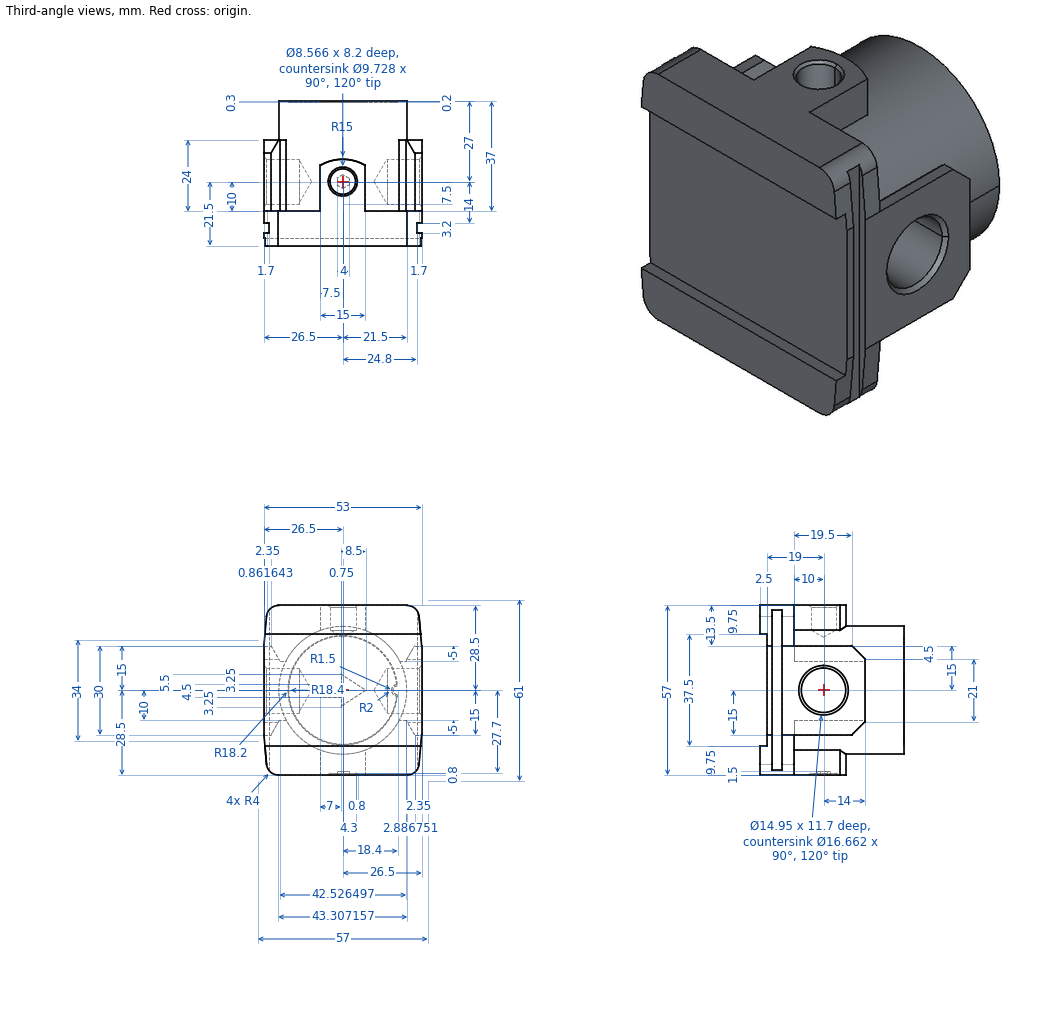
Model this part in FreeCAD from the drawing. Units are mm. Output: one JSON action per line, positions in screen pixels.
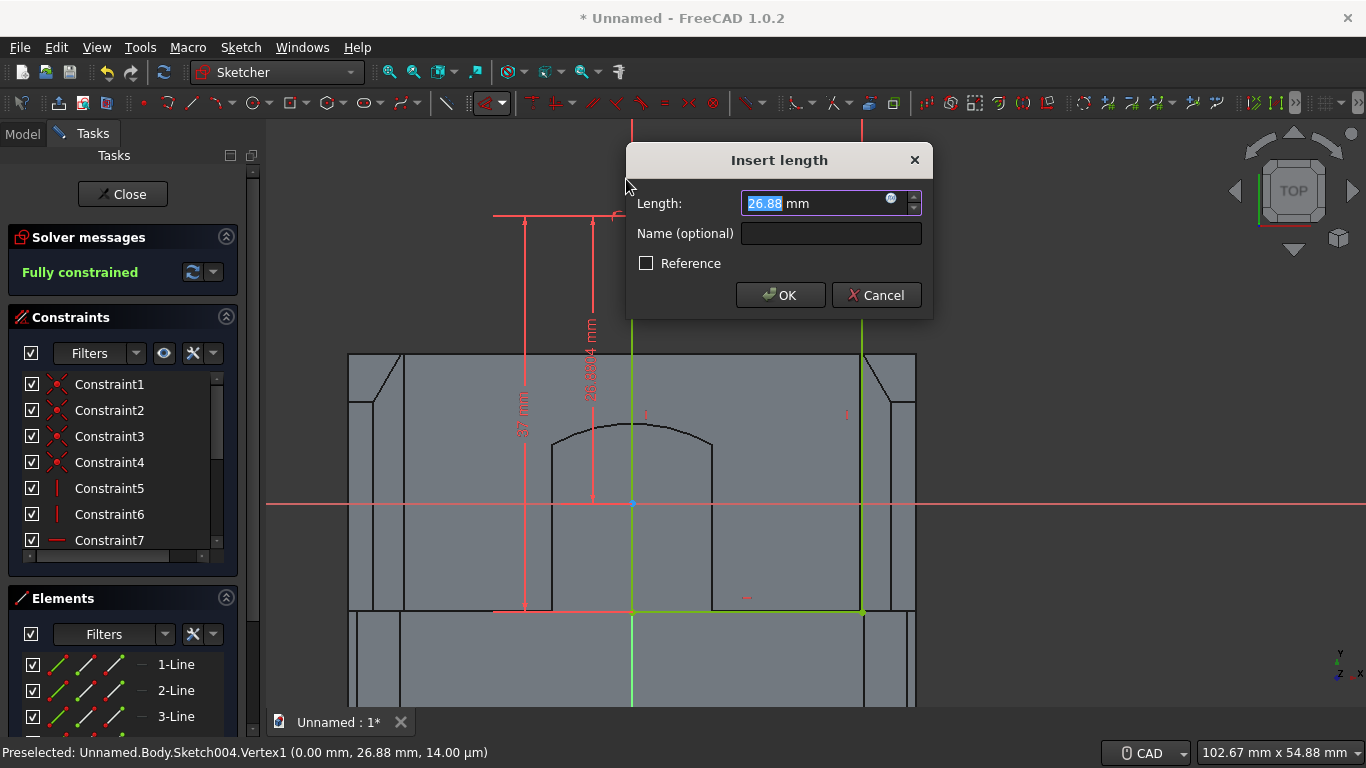
{"action": "type", "text": "27"}
{"action": "key", "text": "Return"}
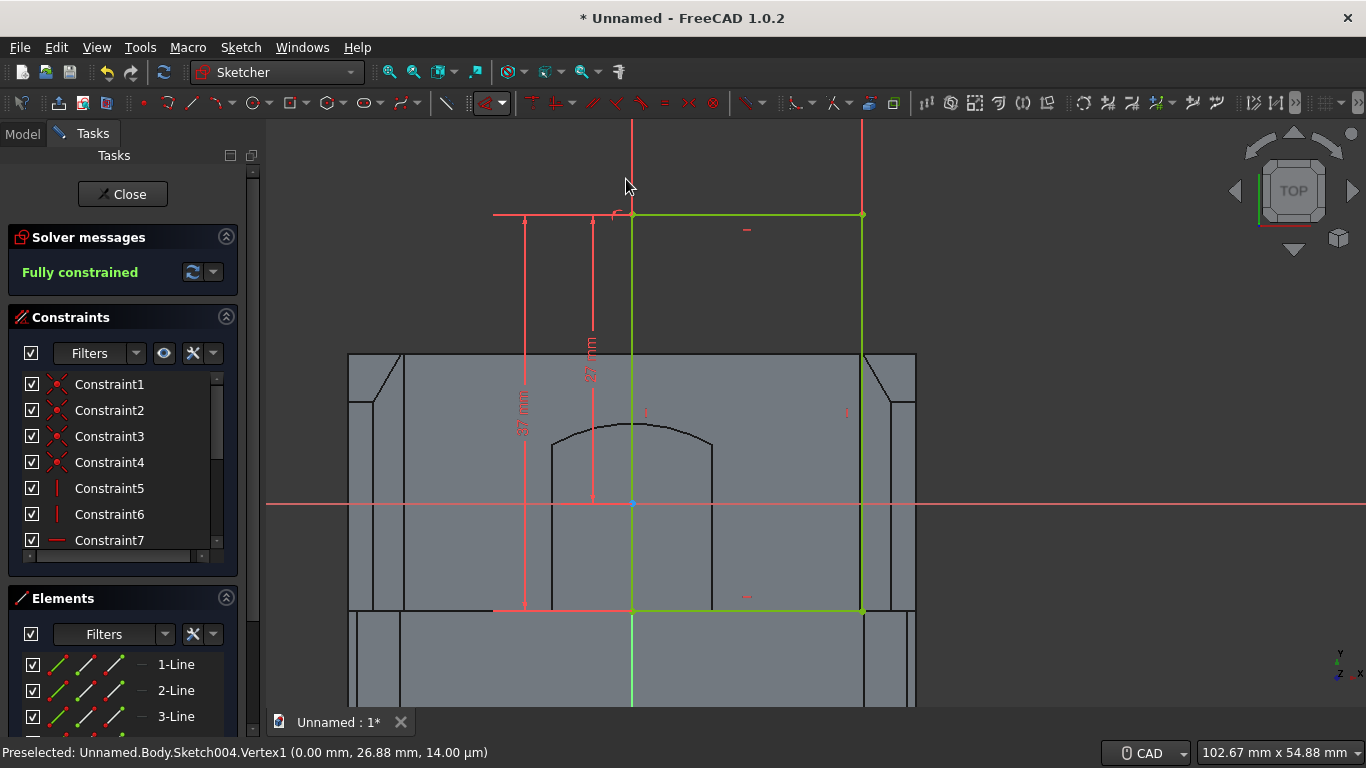
{"action": "left_click", "coordinate": [123, 194]}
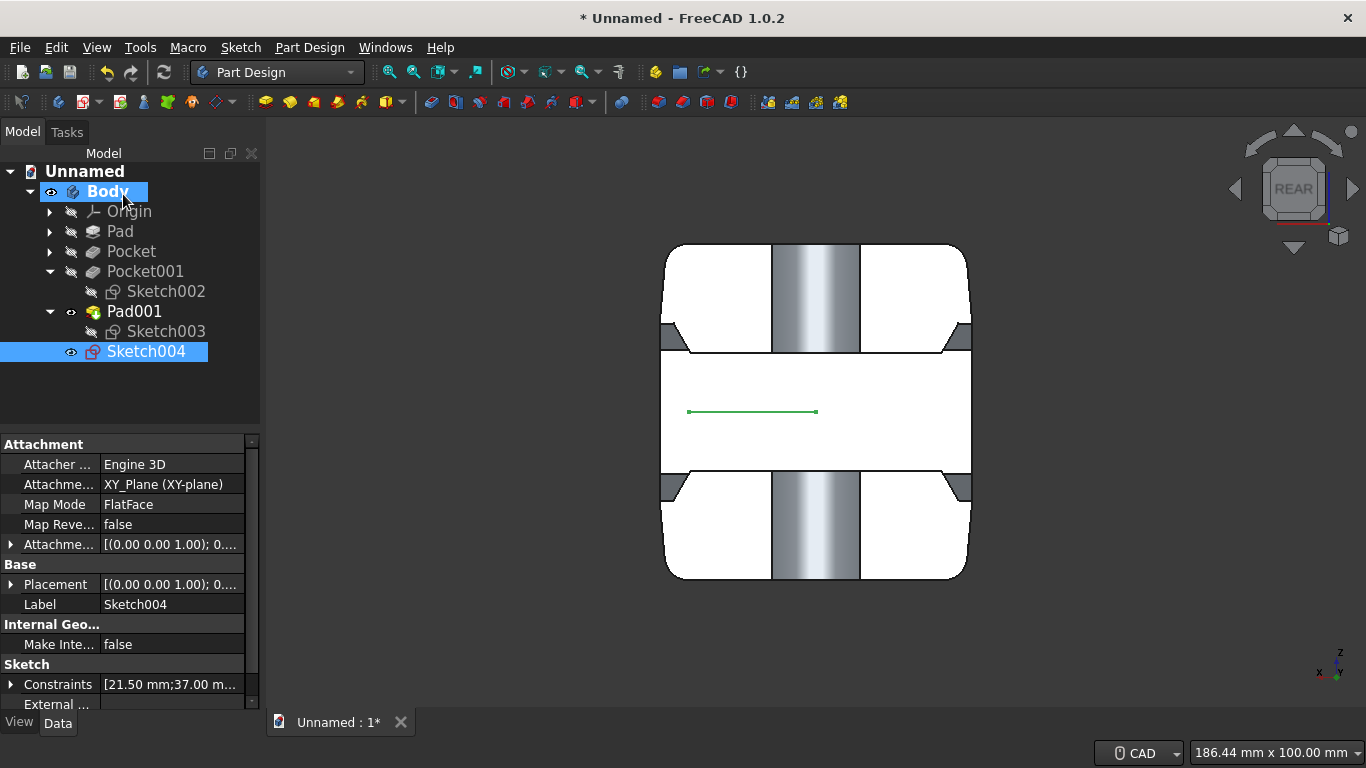
{"action": "left_click", "coordinate": [290, 102]}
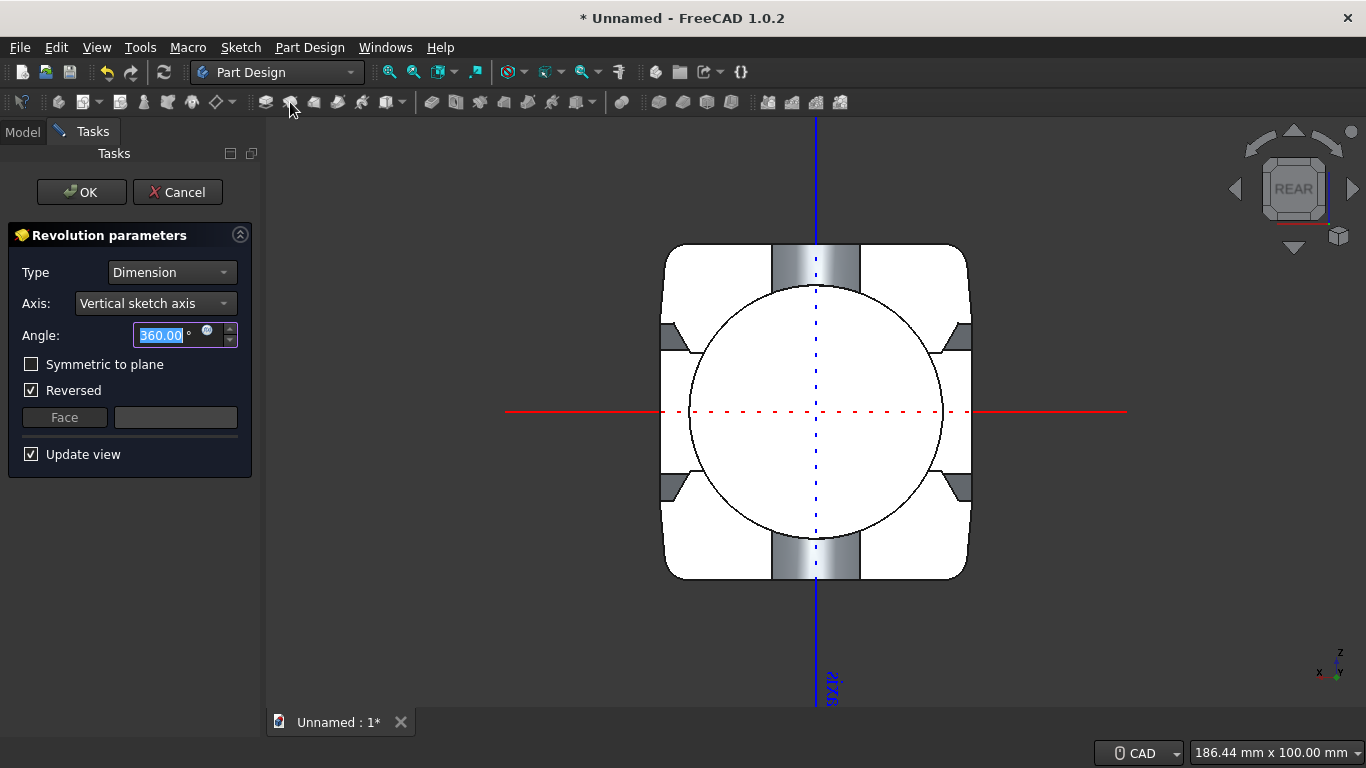
{"action": "left_click", "coordinate": [82, 192]}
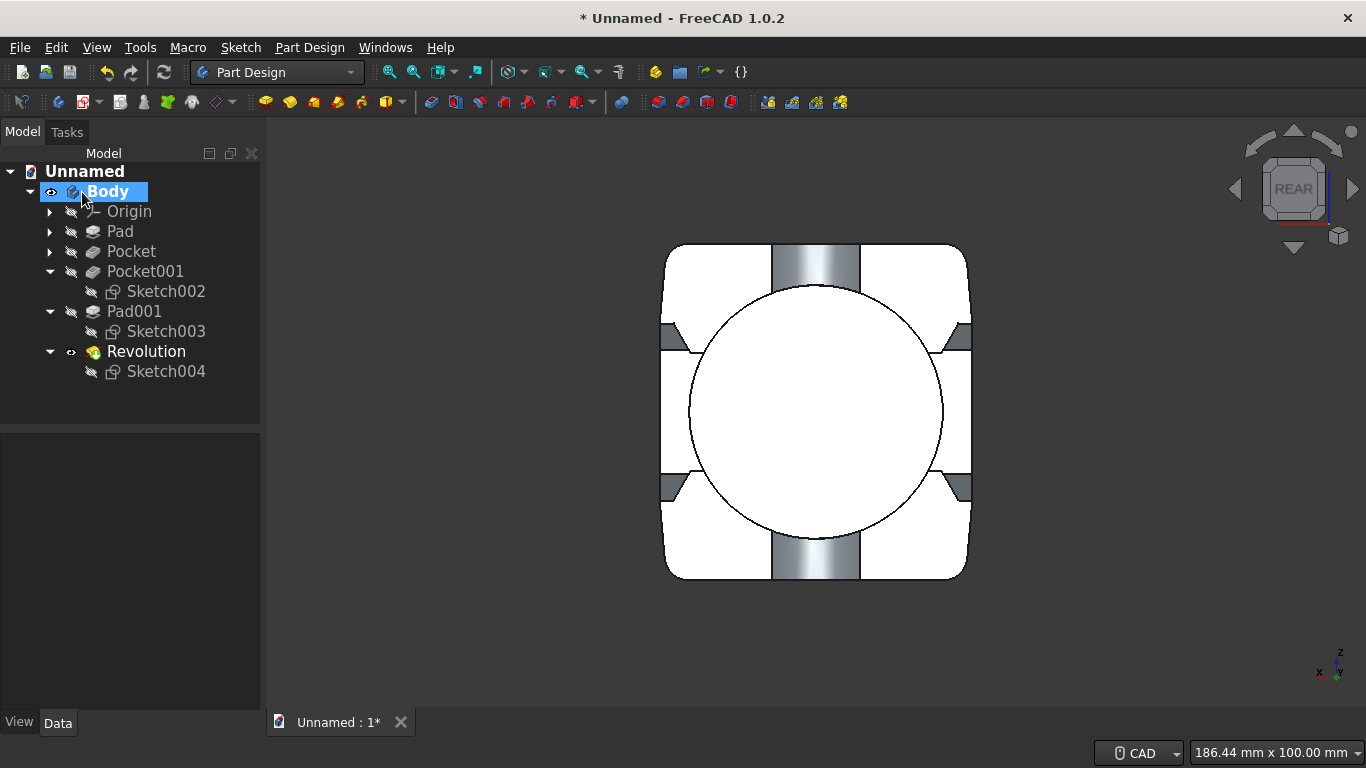
{"action": "left_click", "coordinate": [84, 102]}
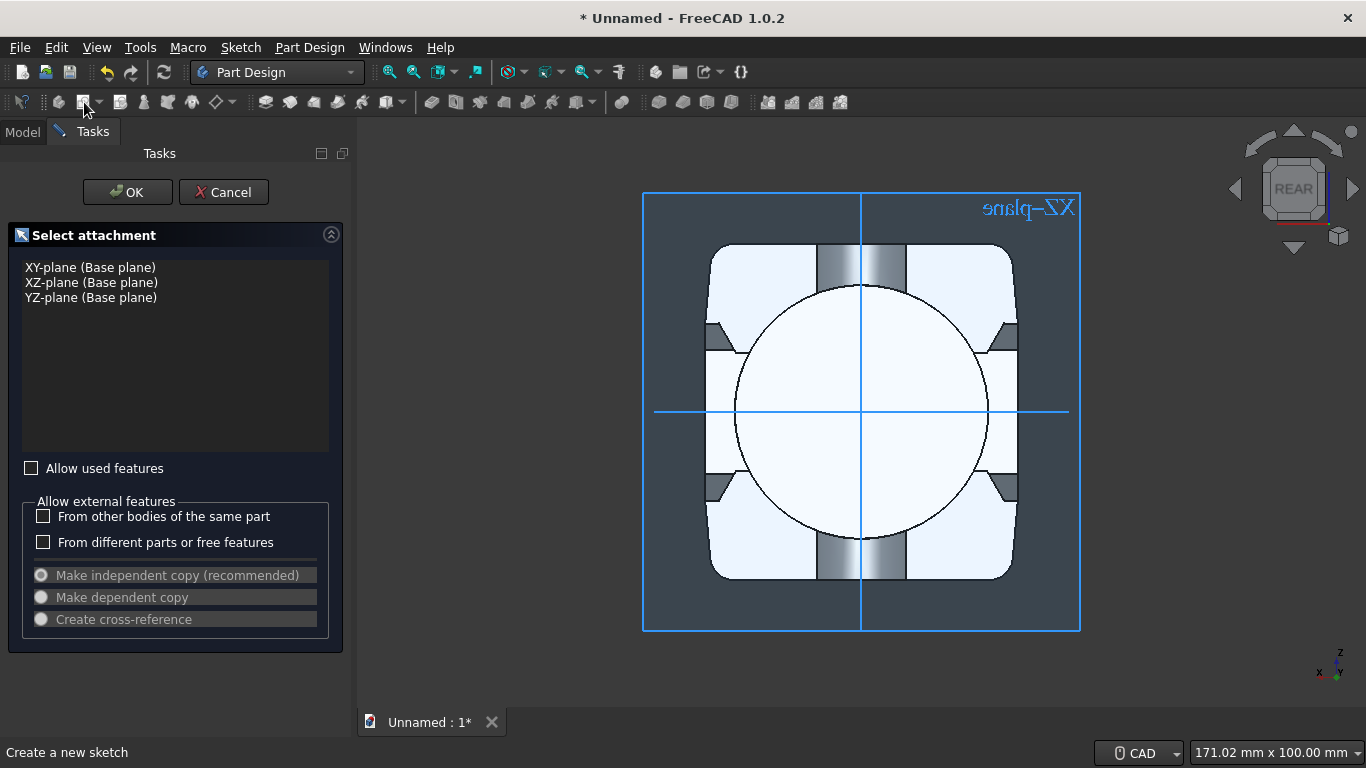
{"action": "left_click", "coordinate": [82, 268]}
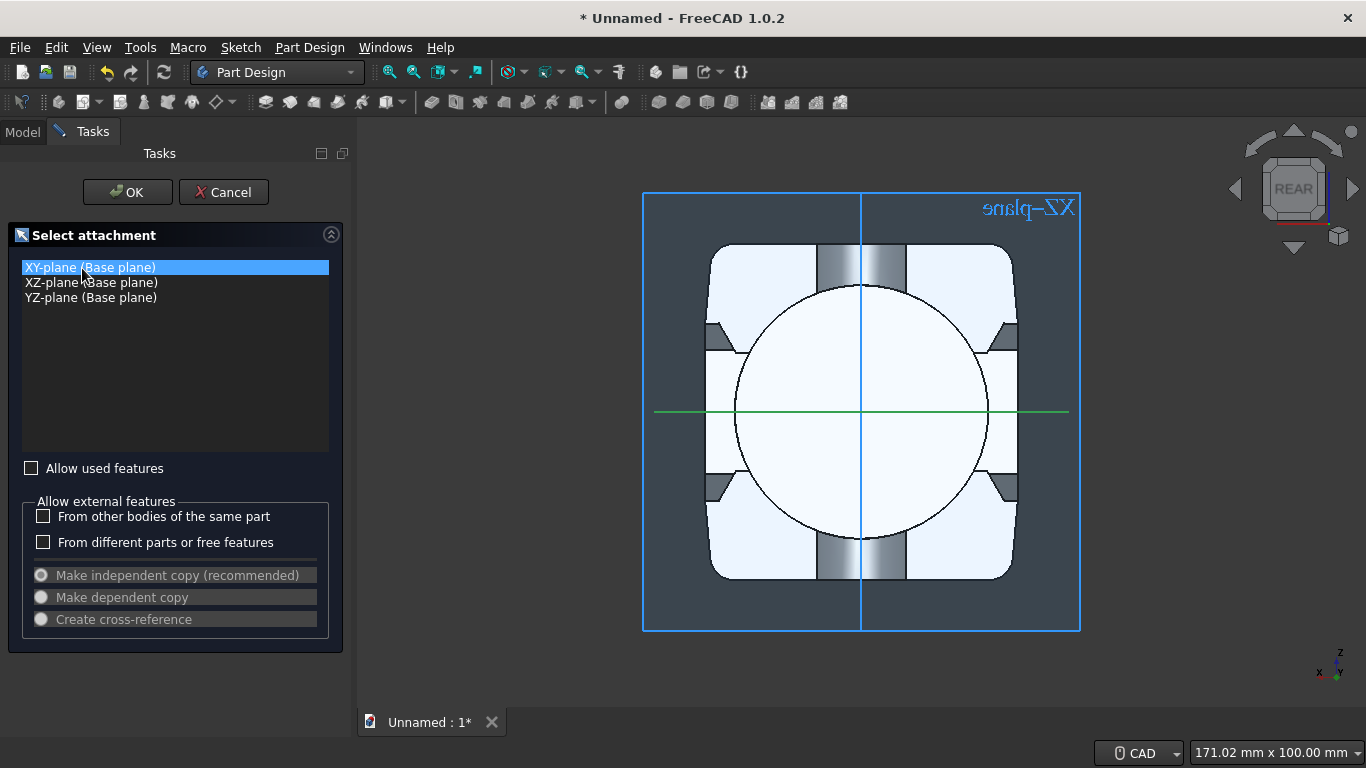
{"action": "left_click", "coordinate": [128, 192]}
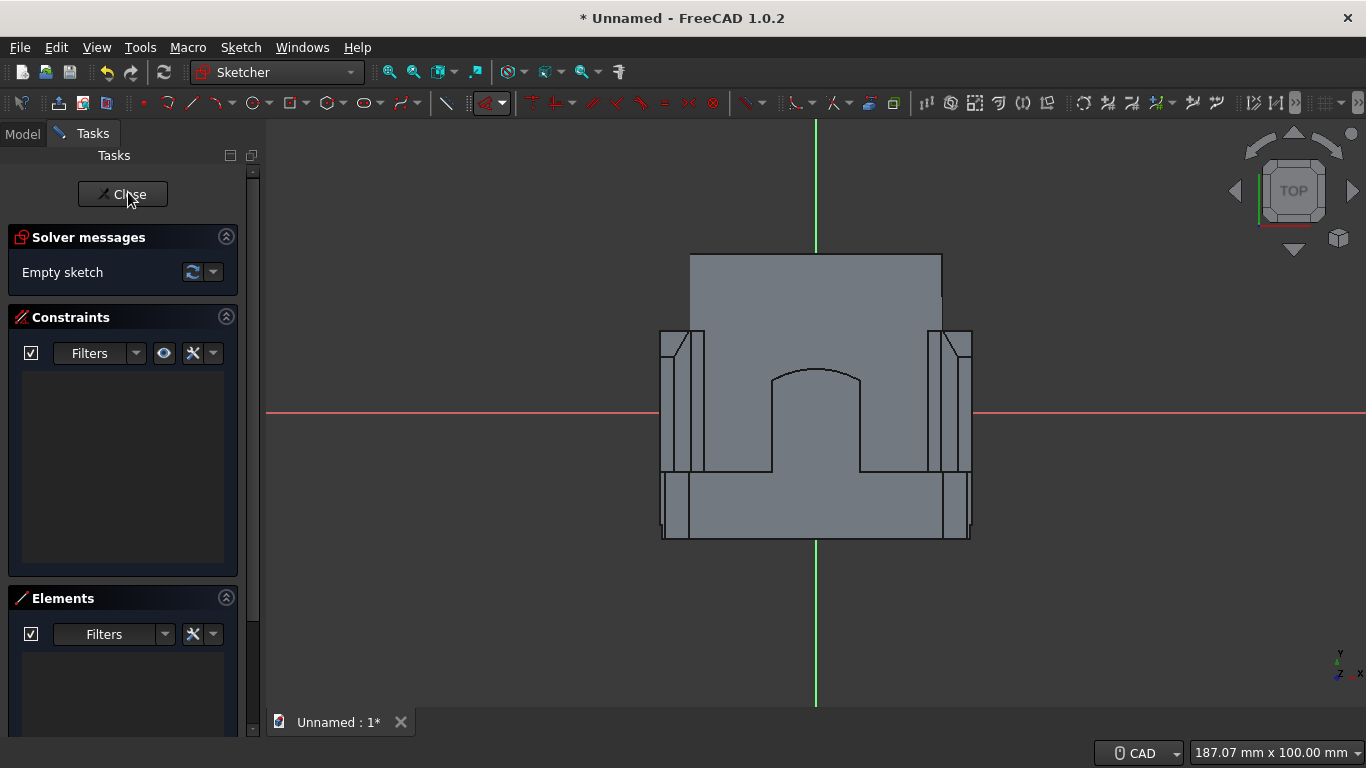
{"action": "left_click", "coordinate": [108, 104]}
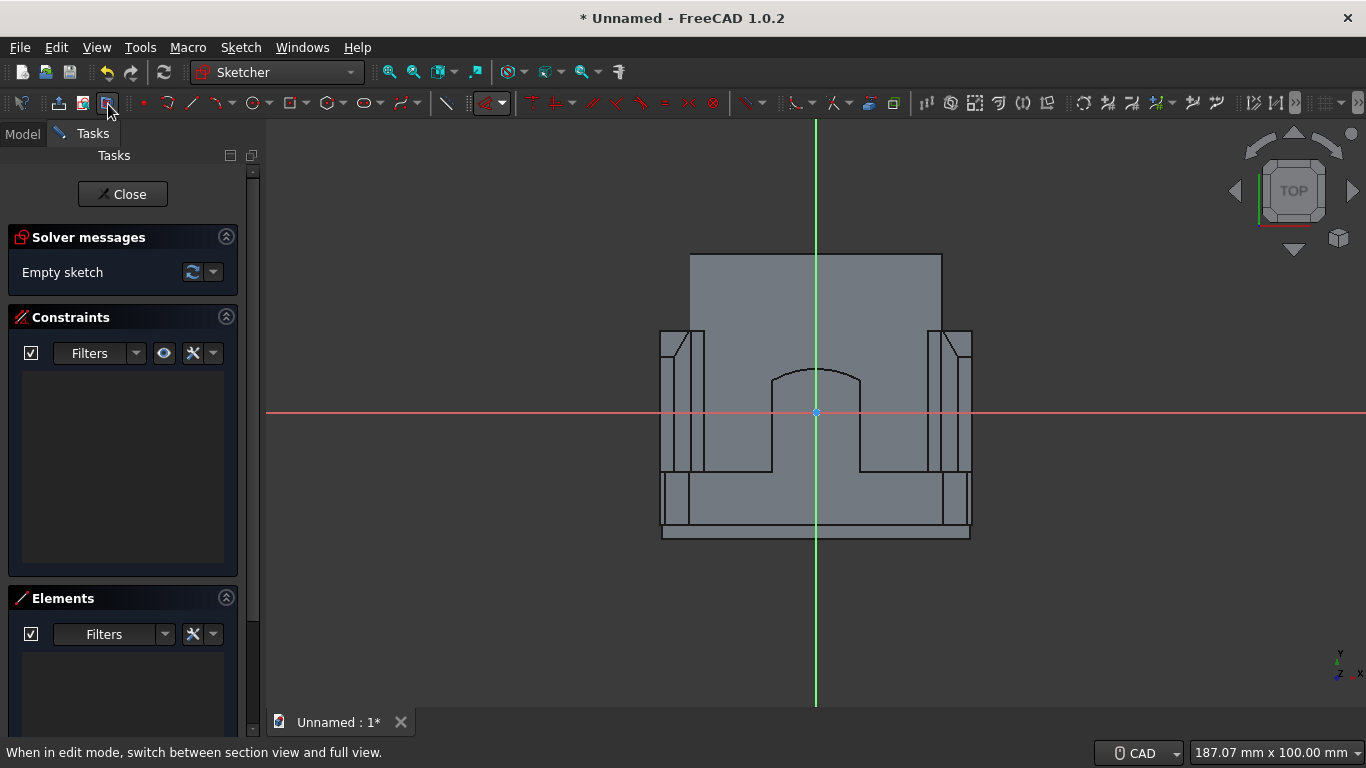
{"action": "scroll", "coordinate": [978, 510], "scroll_direction": "up", "scroll_amount": 15}